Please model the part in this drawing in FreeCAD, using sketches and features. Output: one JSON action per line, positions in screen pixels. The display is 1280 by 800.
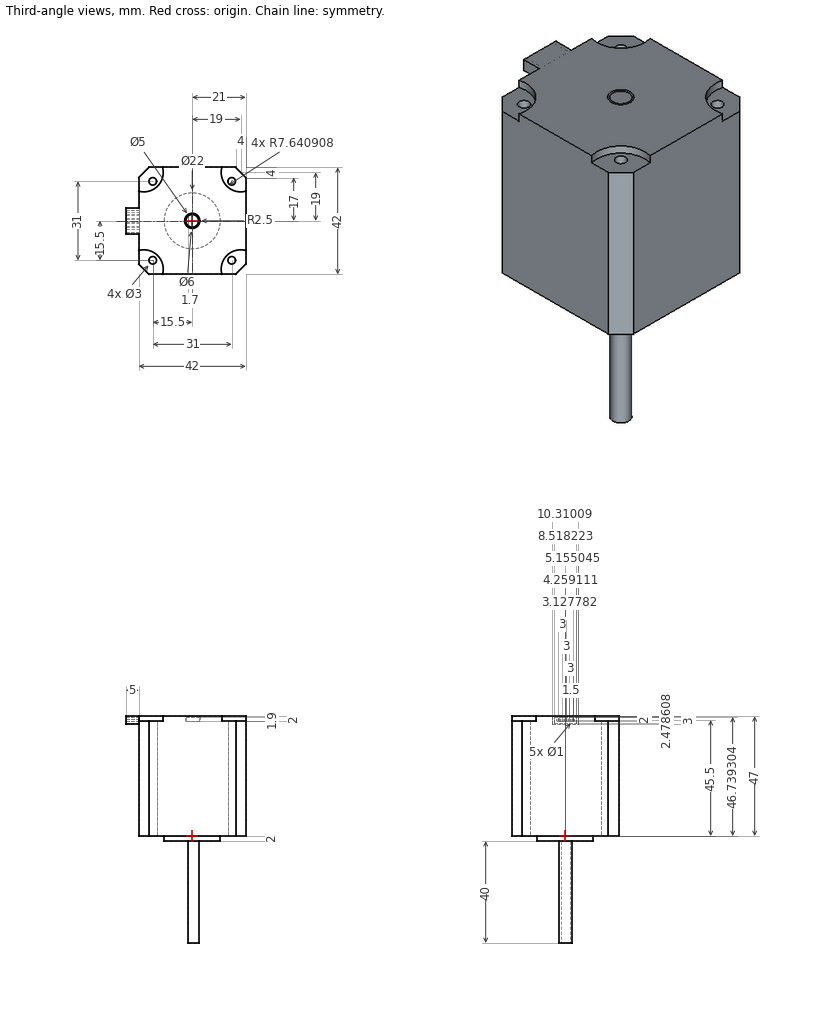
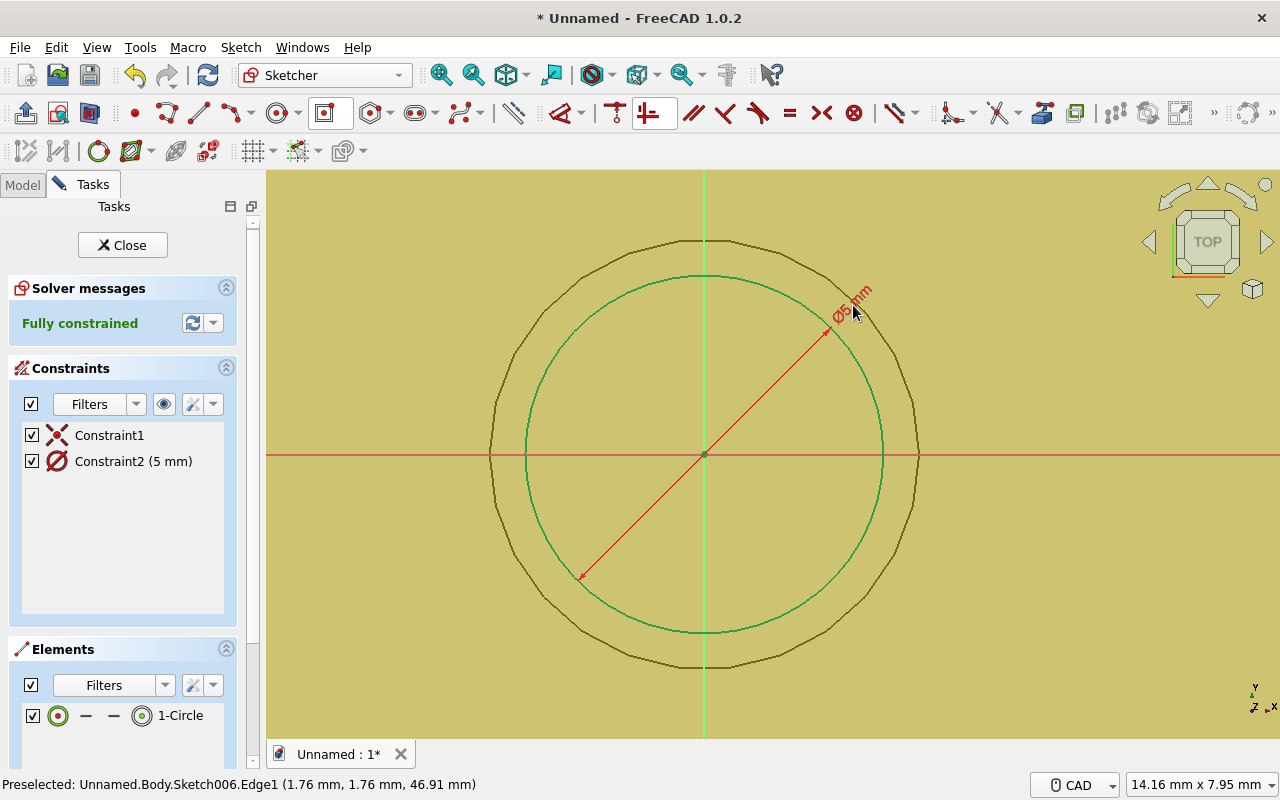
{"action": "left_click", "coordinate": [123, 245]}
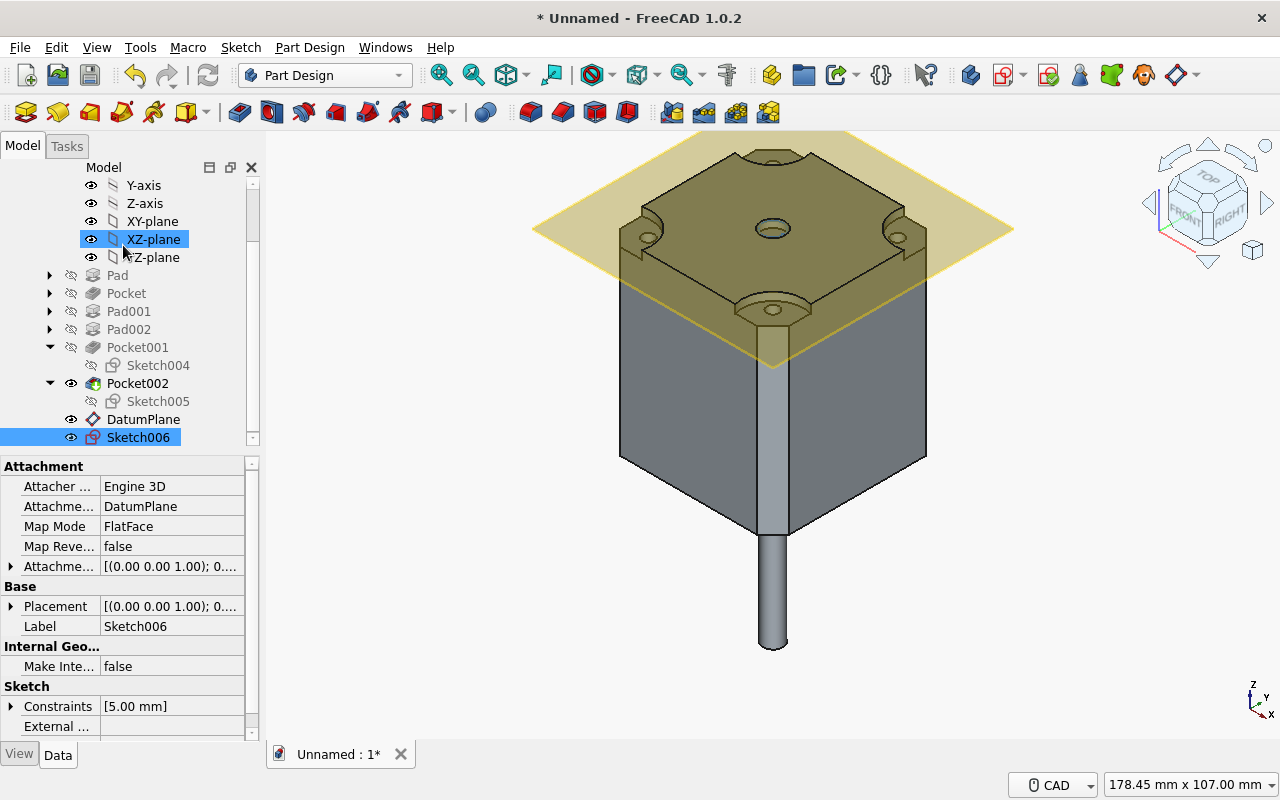
{"action": "left_click", "coordinate": [26, 112]}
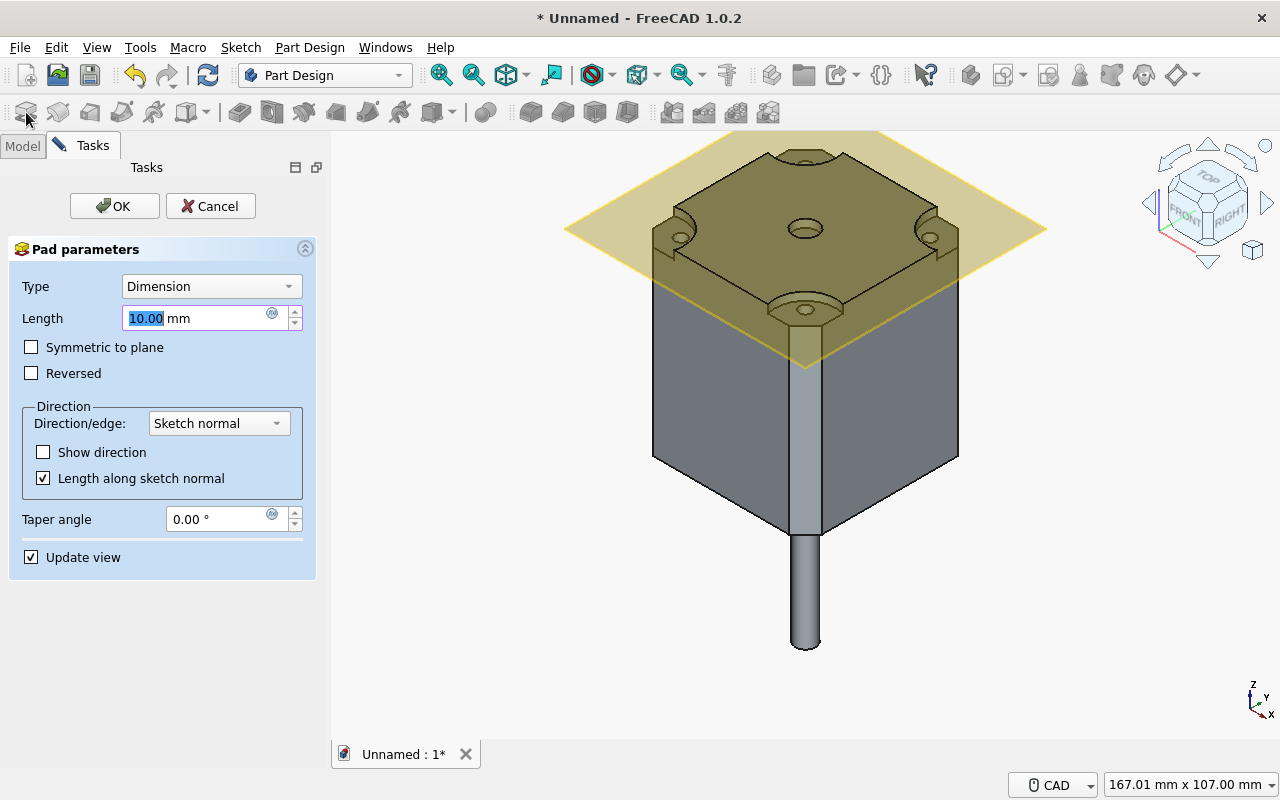
{"action": "type", "text": "1.9"}
{"action": "key", "text": "Tab"}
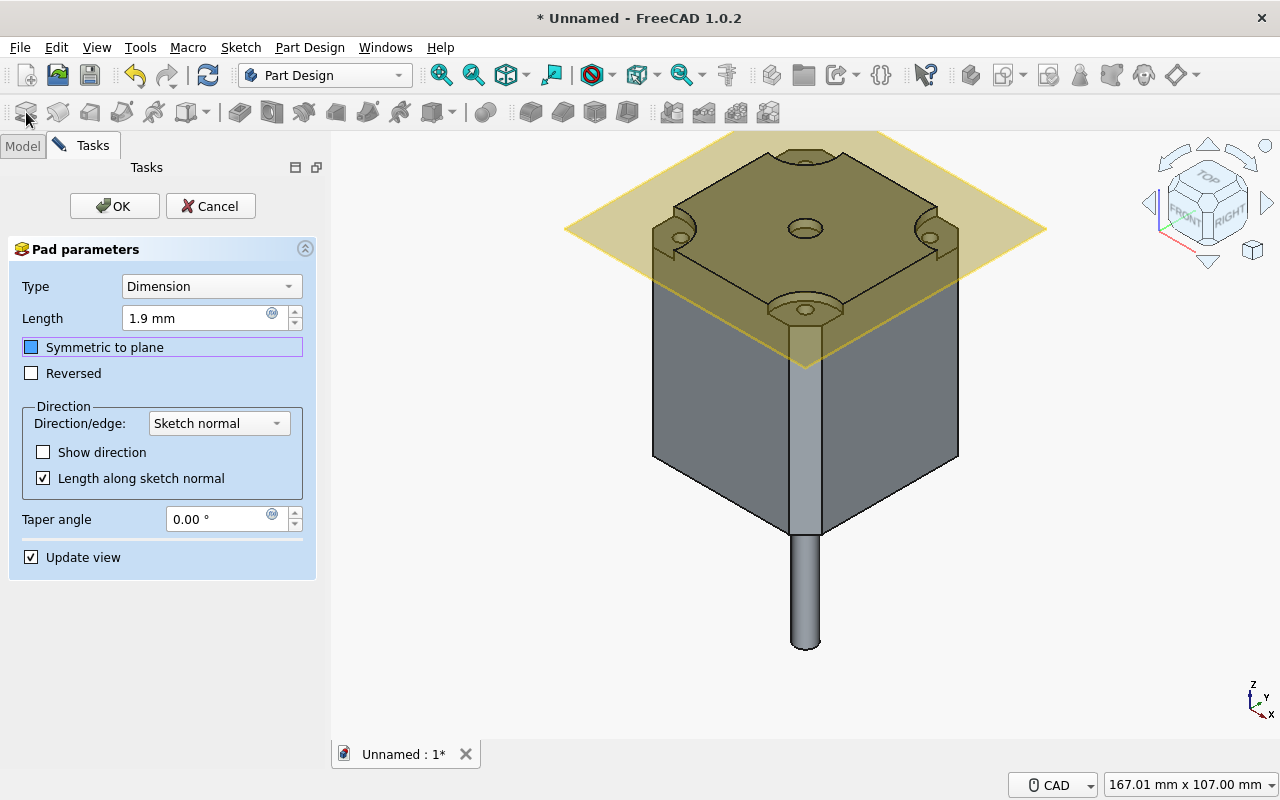
{"action": "left_click", "coordinate": [30, 373]}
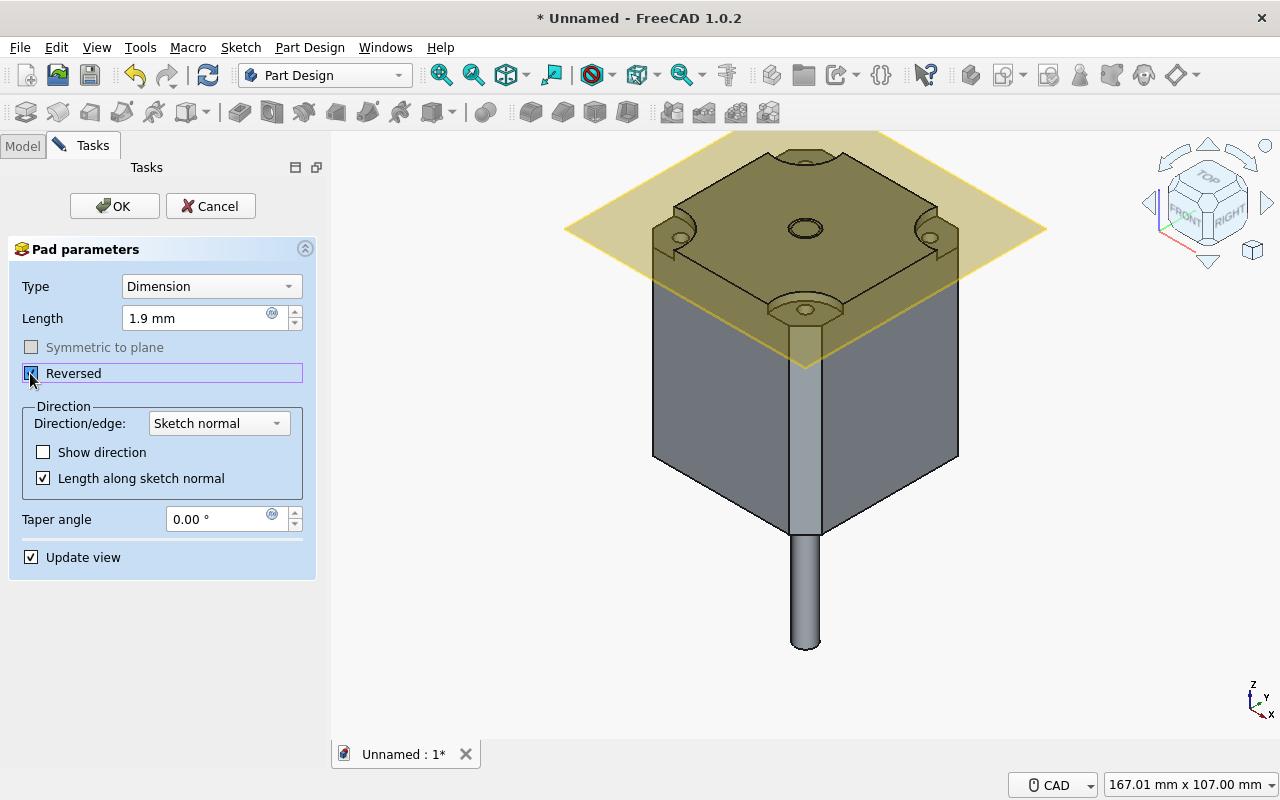
{"action": "left_click", "coordinate": [115, 206]}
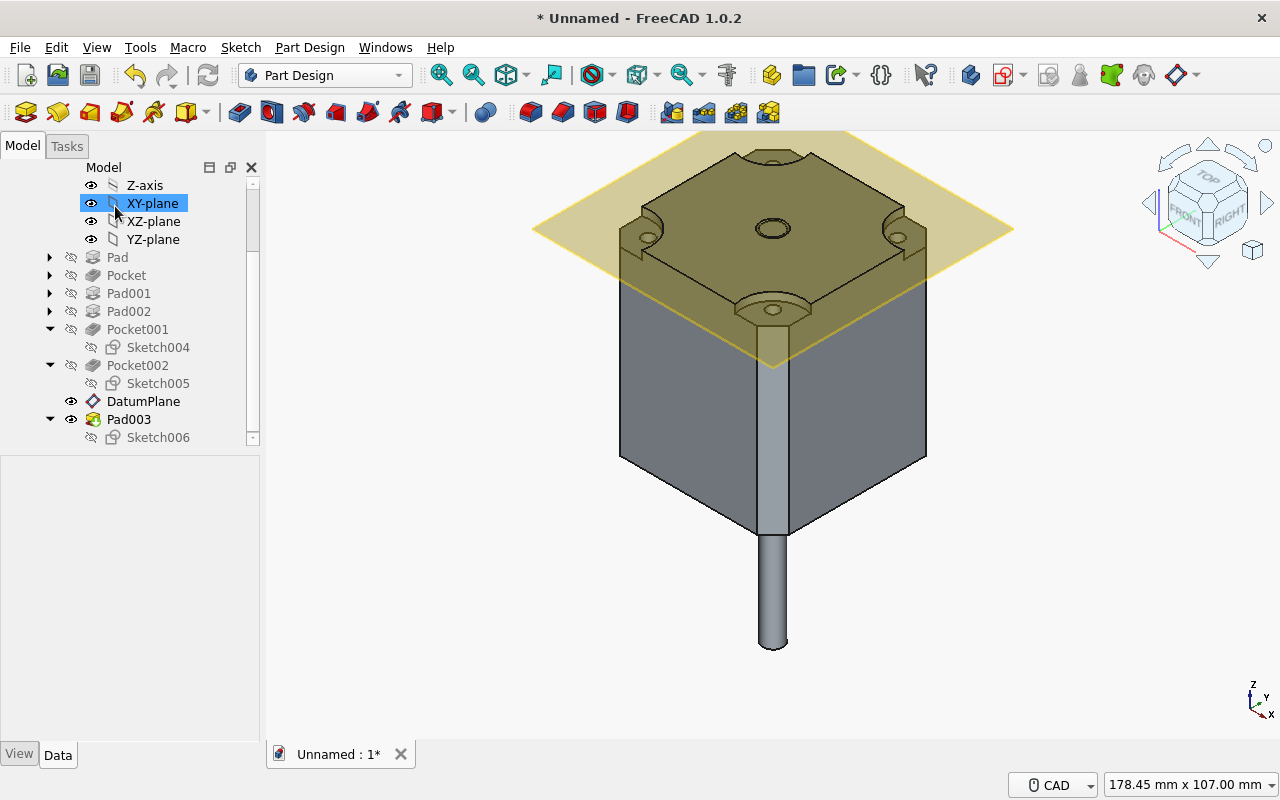
{"action": "left_click", "coordinate": [116, 401]}
{"action": "key", "text": "space"}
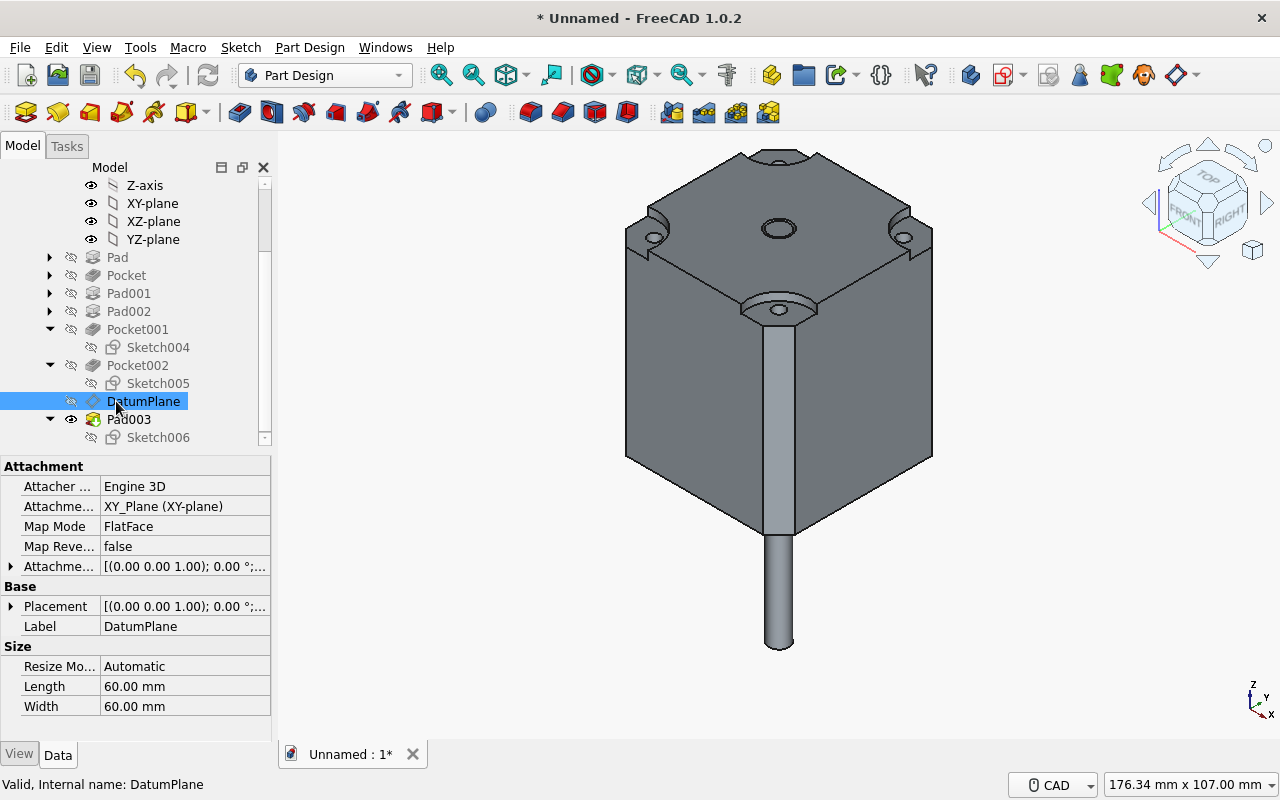
{"action": "left_click", "coordinate": [442, 76]}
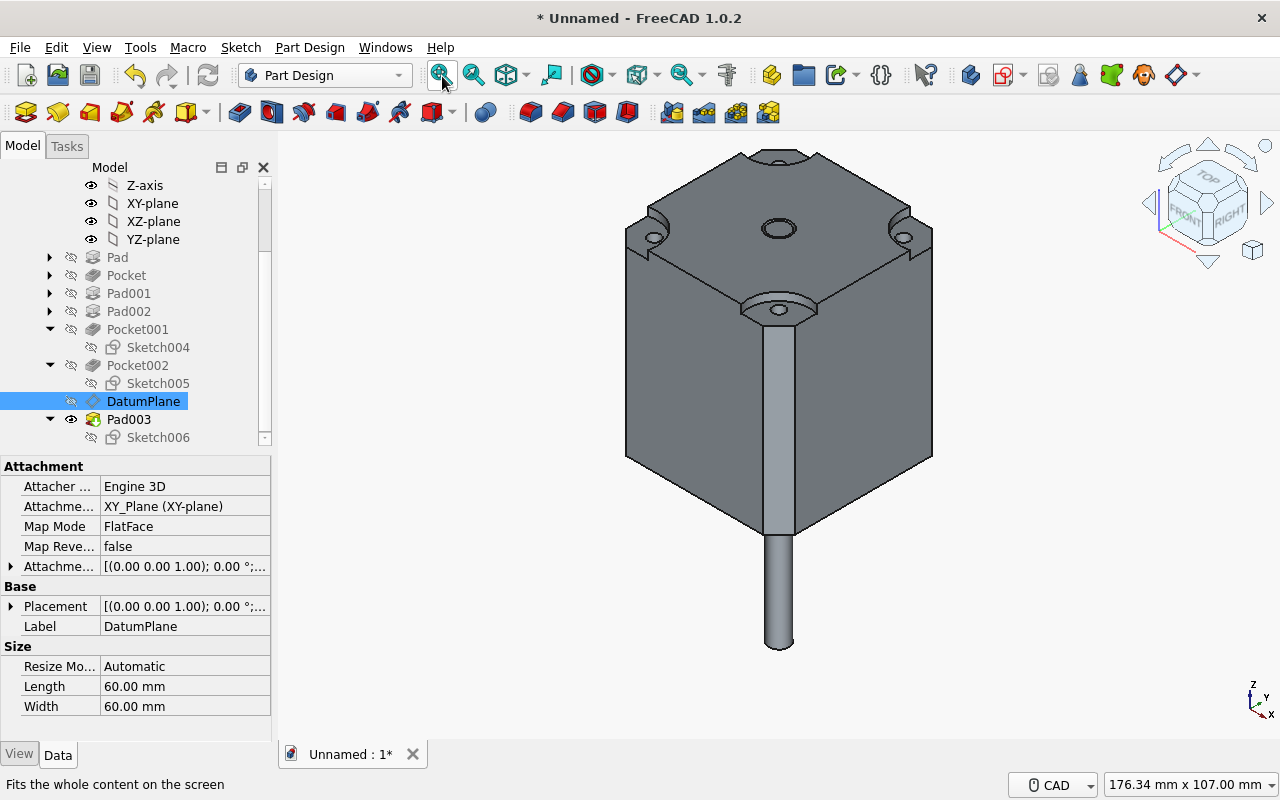
{"action": "key", "text": "6"}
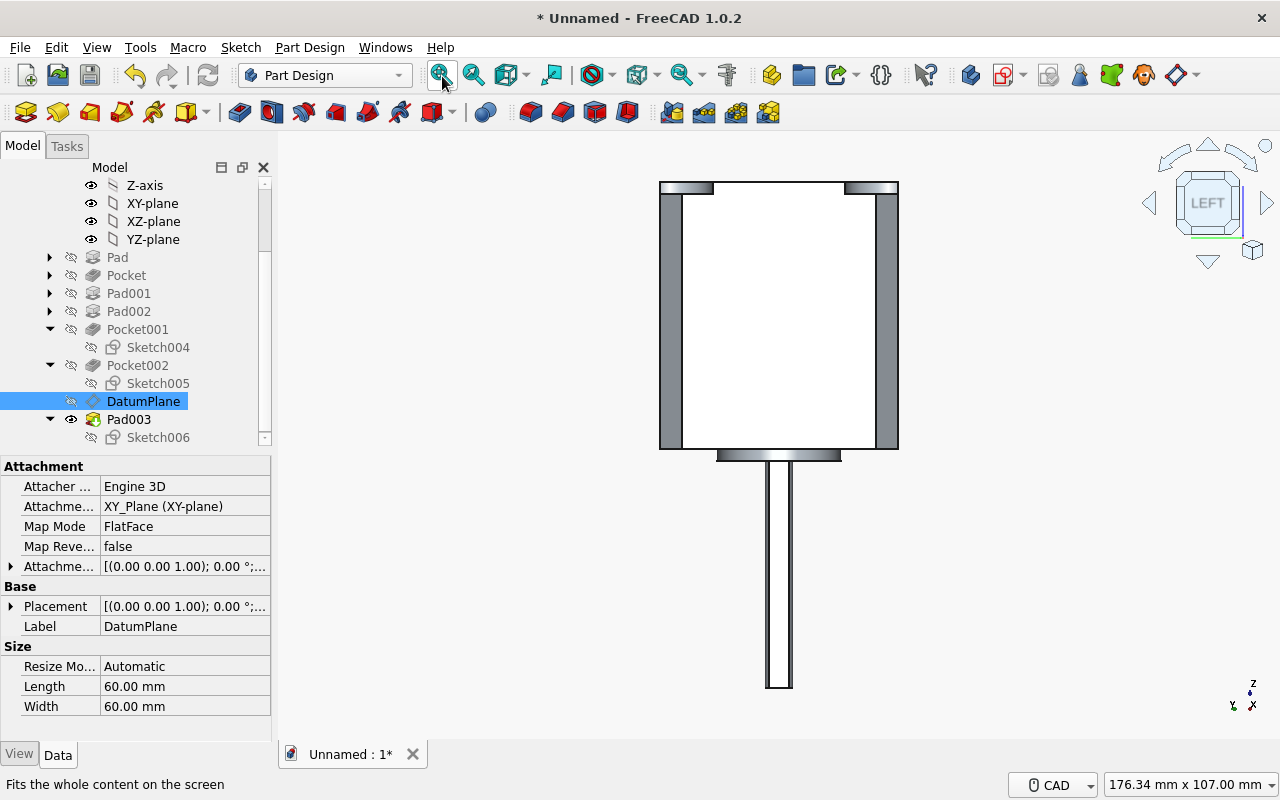
{"action": "left_click", "coordinate": [779, 315]}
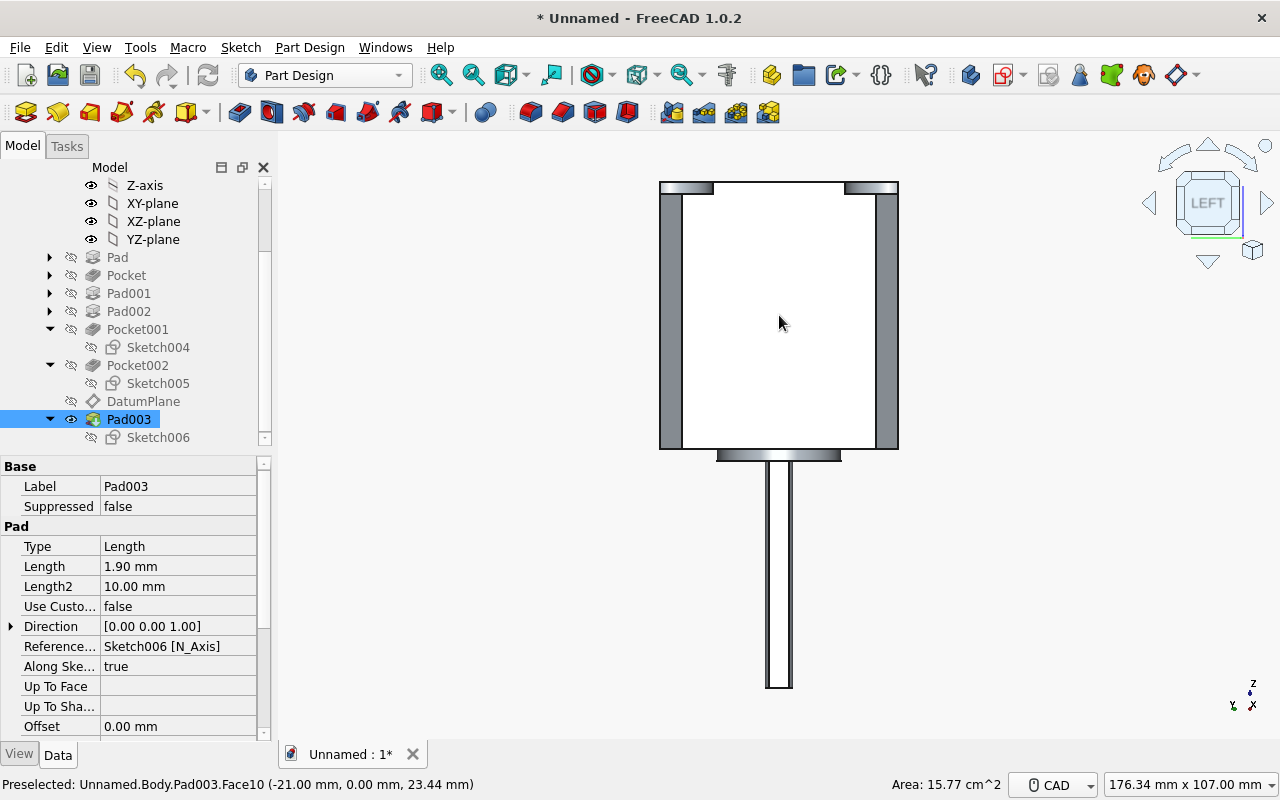
{"action": "left_click", "coordinate": [1004, 76]}